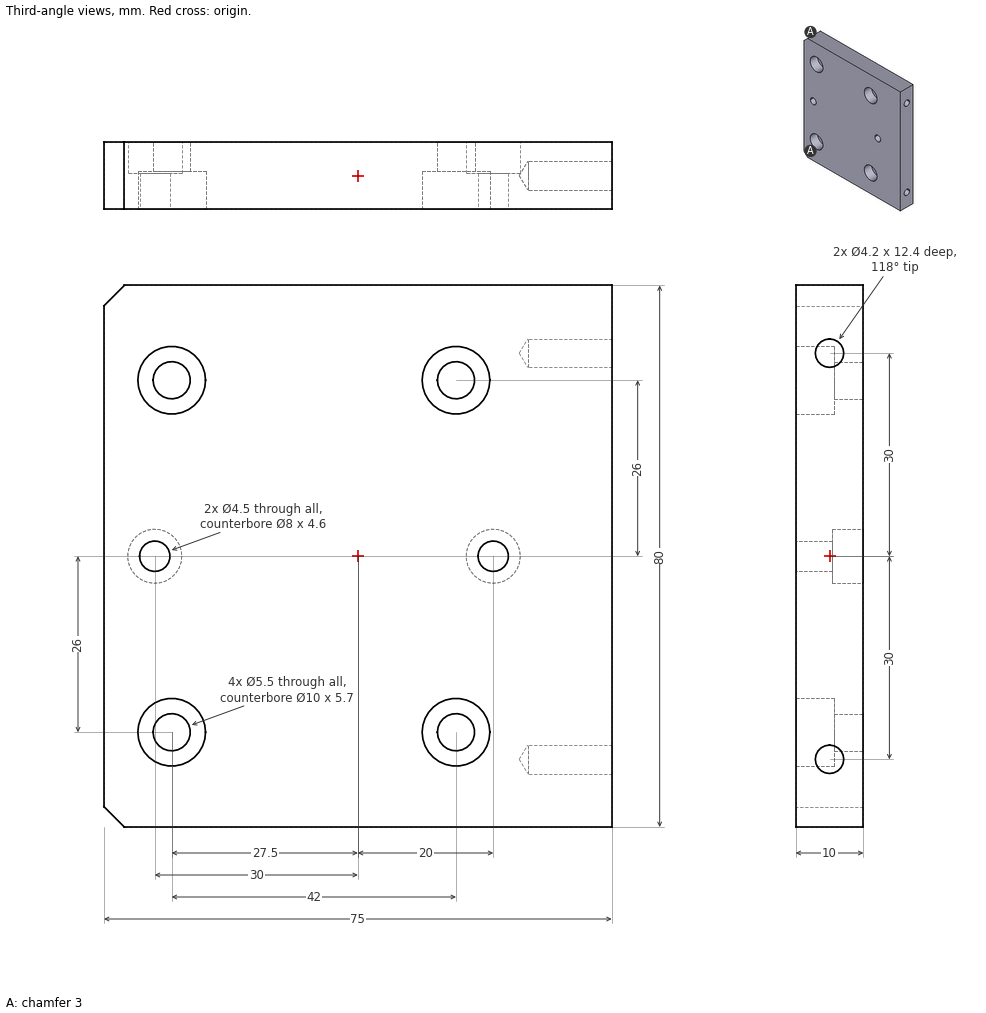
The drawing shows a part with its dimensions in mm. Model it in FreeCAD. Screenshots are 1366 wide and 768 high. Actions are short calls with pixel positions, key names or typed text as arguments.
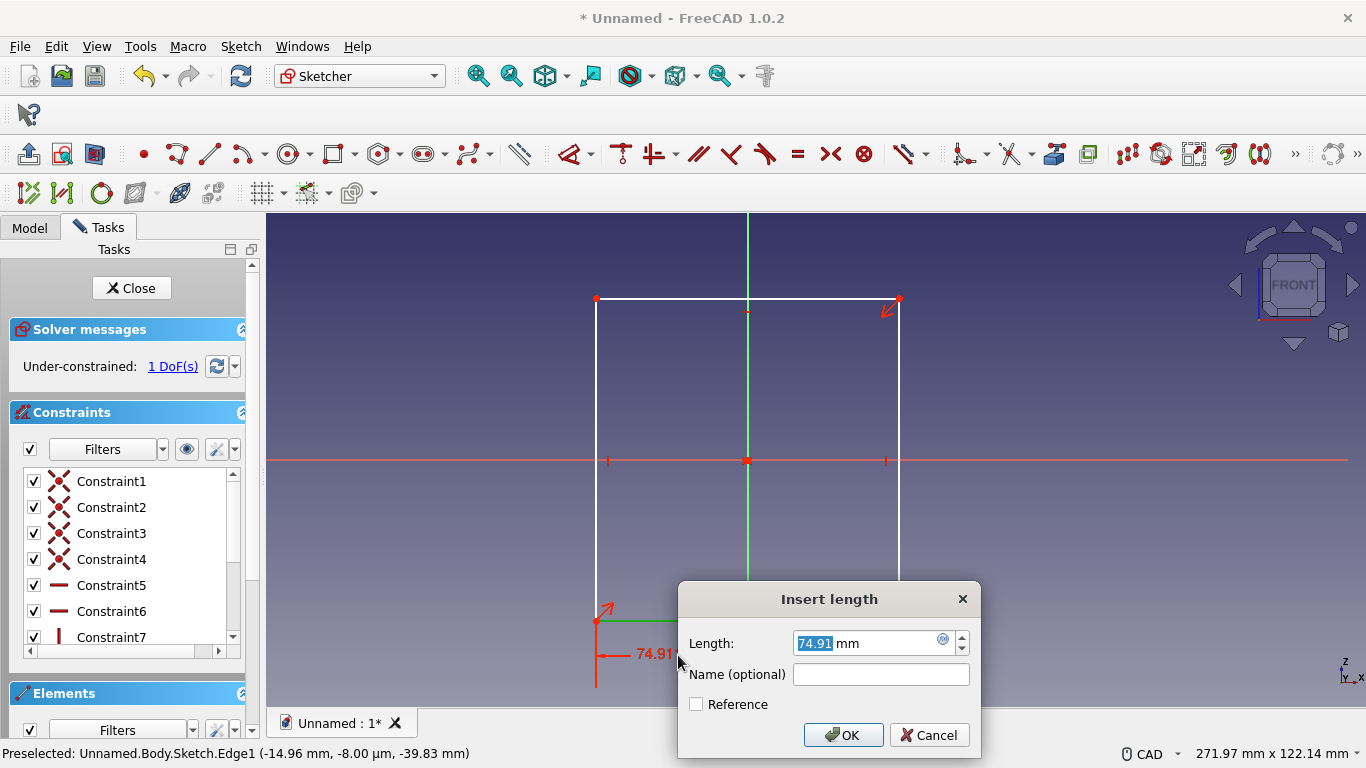
text(75)
key(Return)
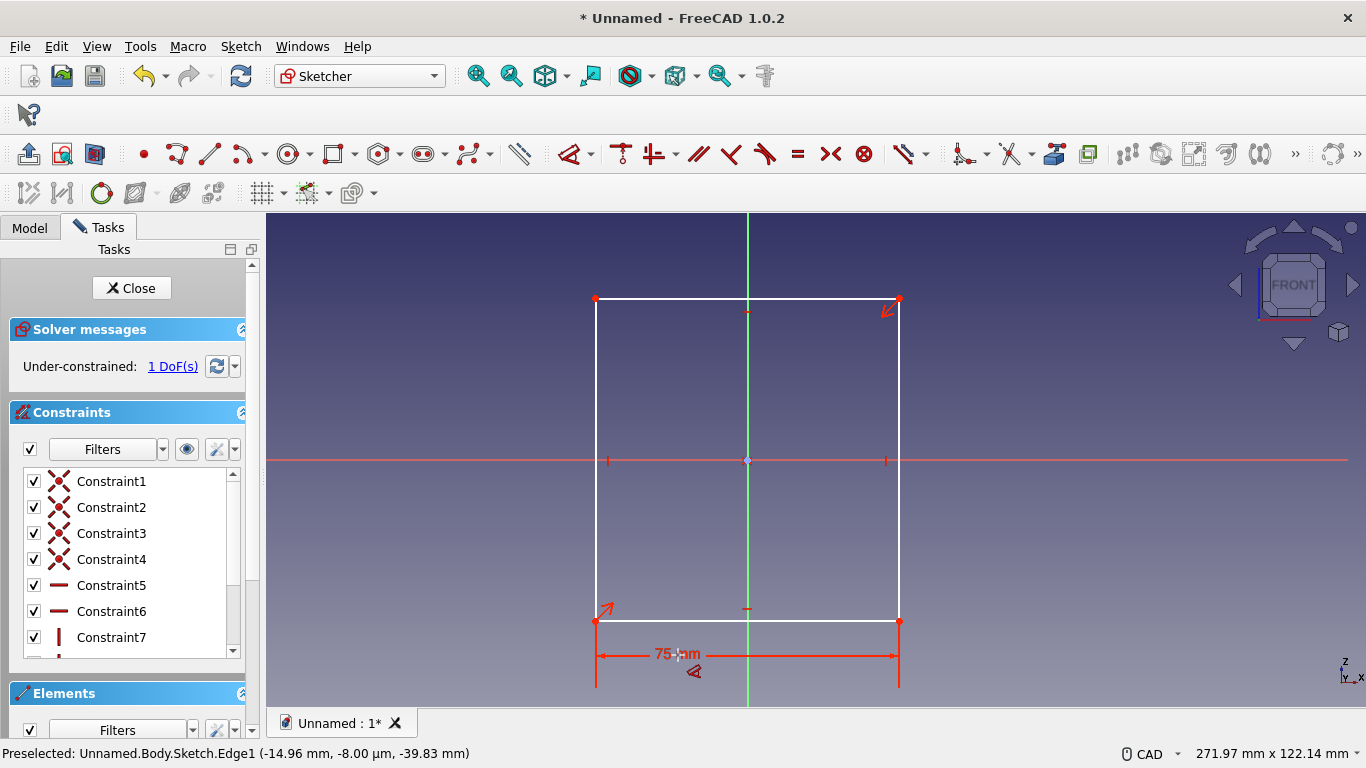
click(899, 525)
click(933, 386)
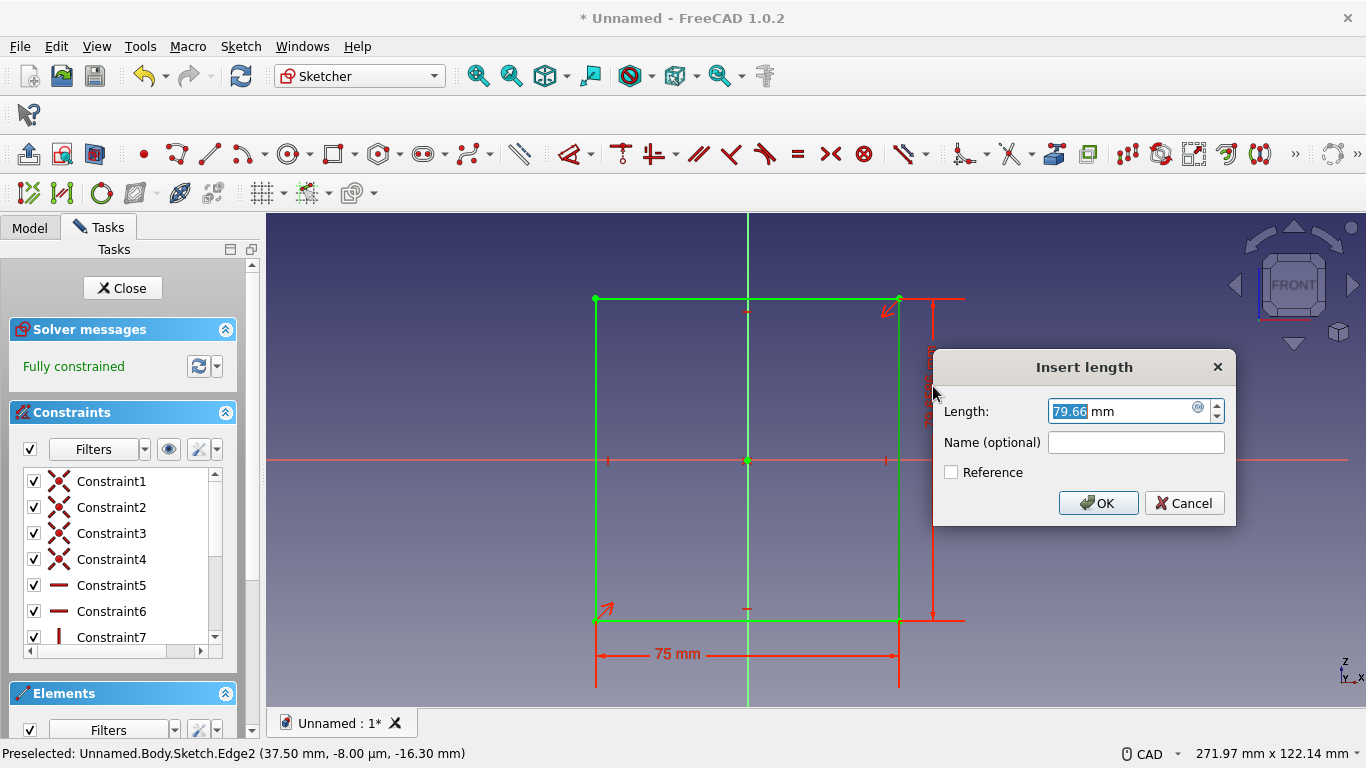
text(80)
key(Return)
key(Escape)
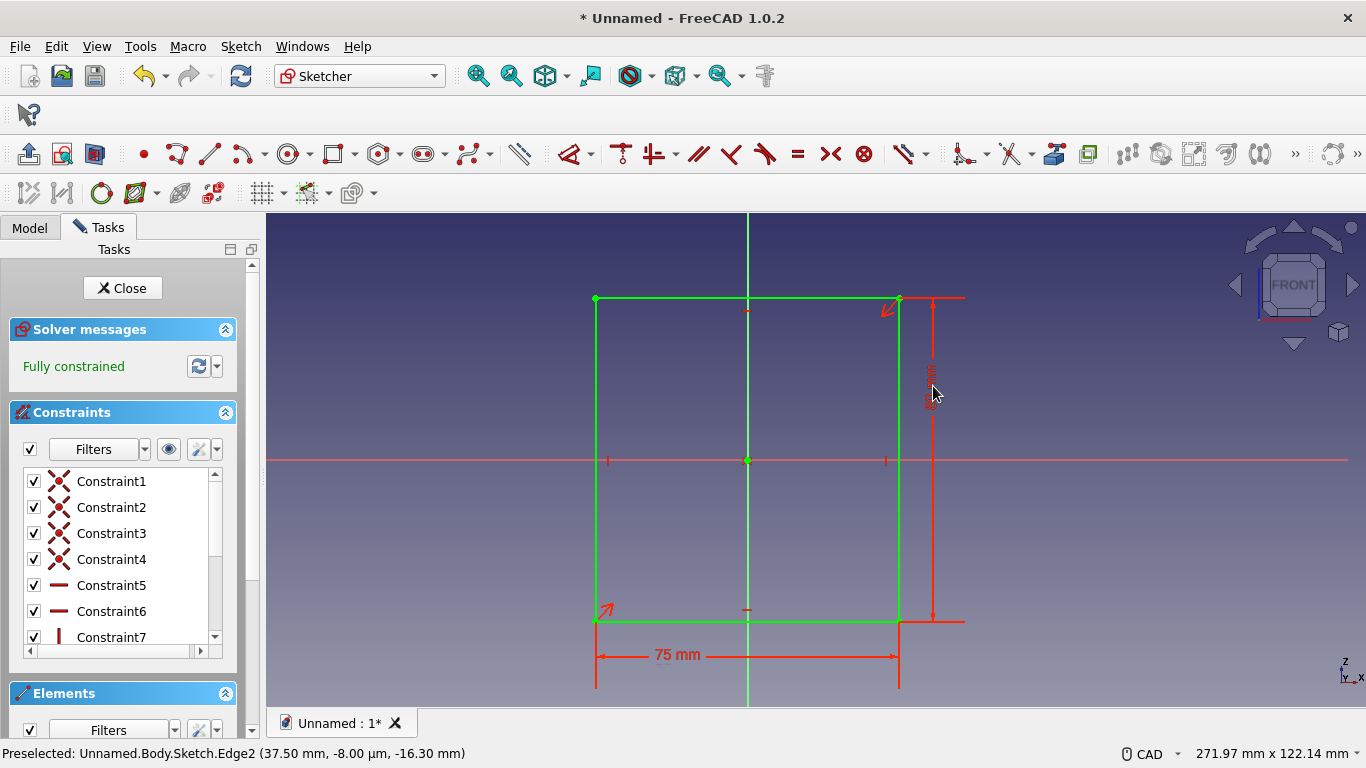
click(123, 288)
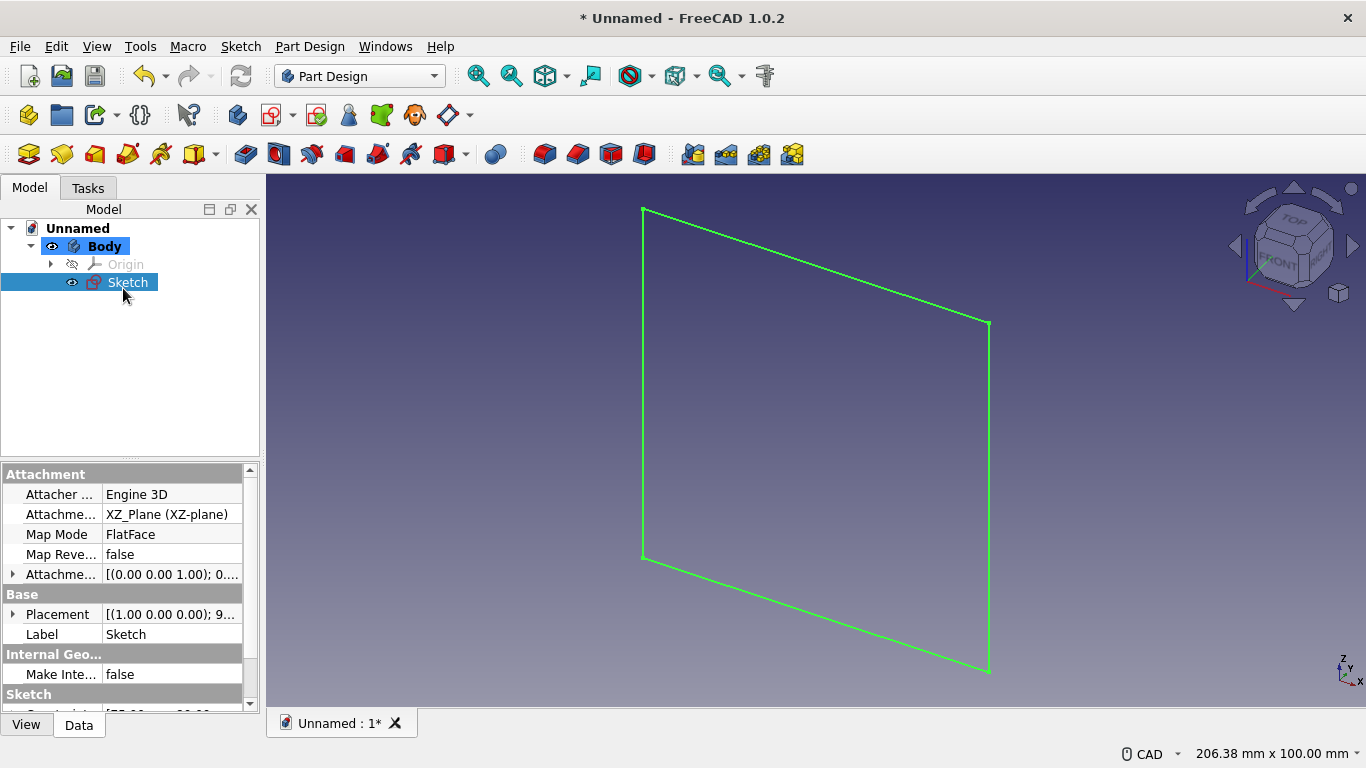
click(29, 154)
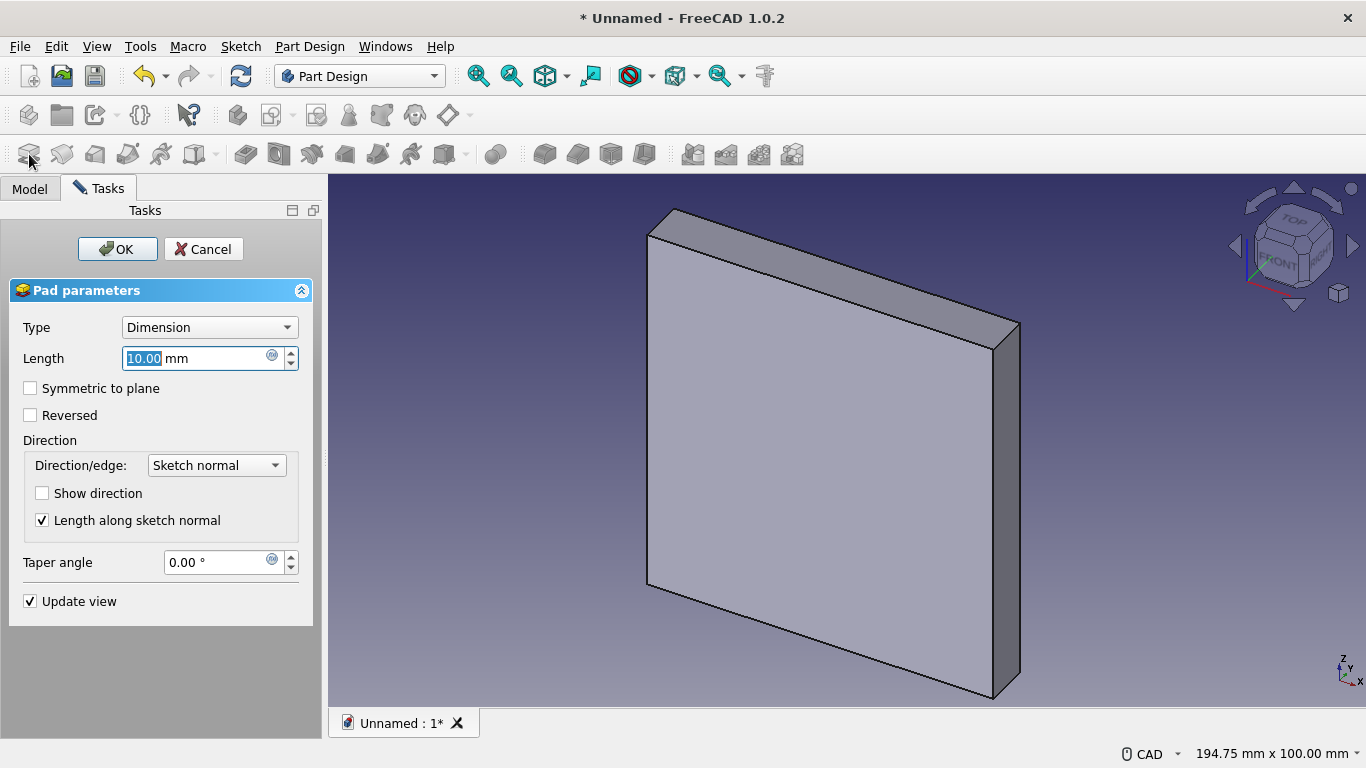
text(10)
key(Tab)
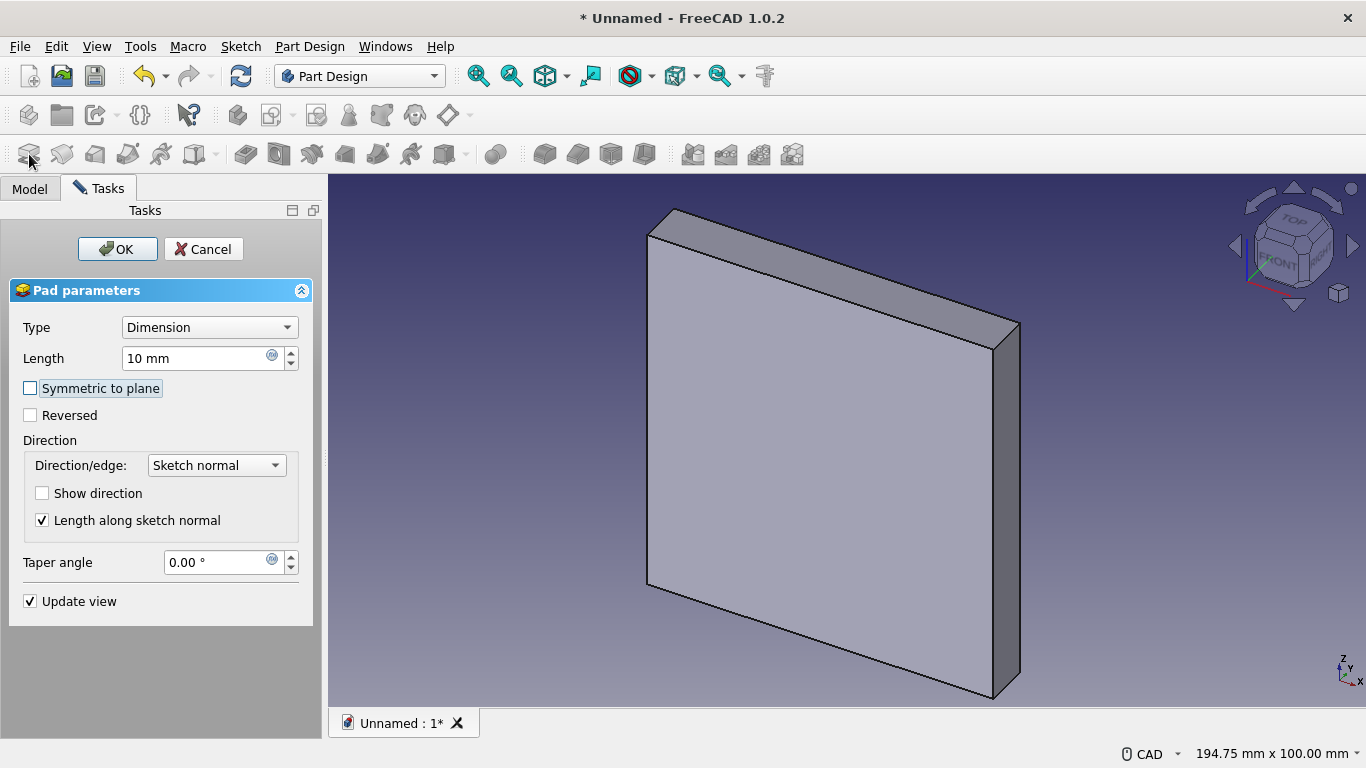
click(31, 388)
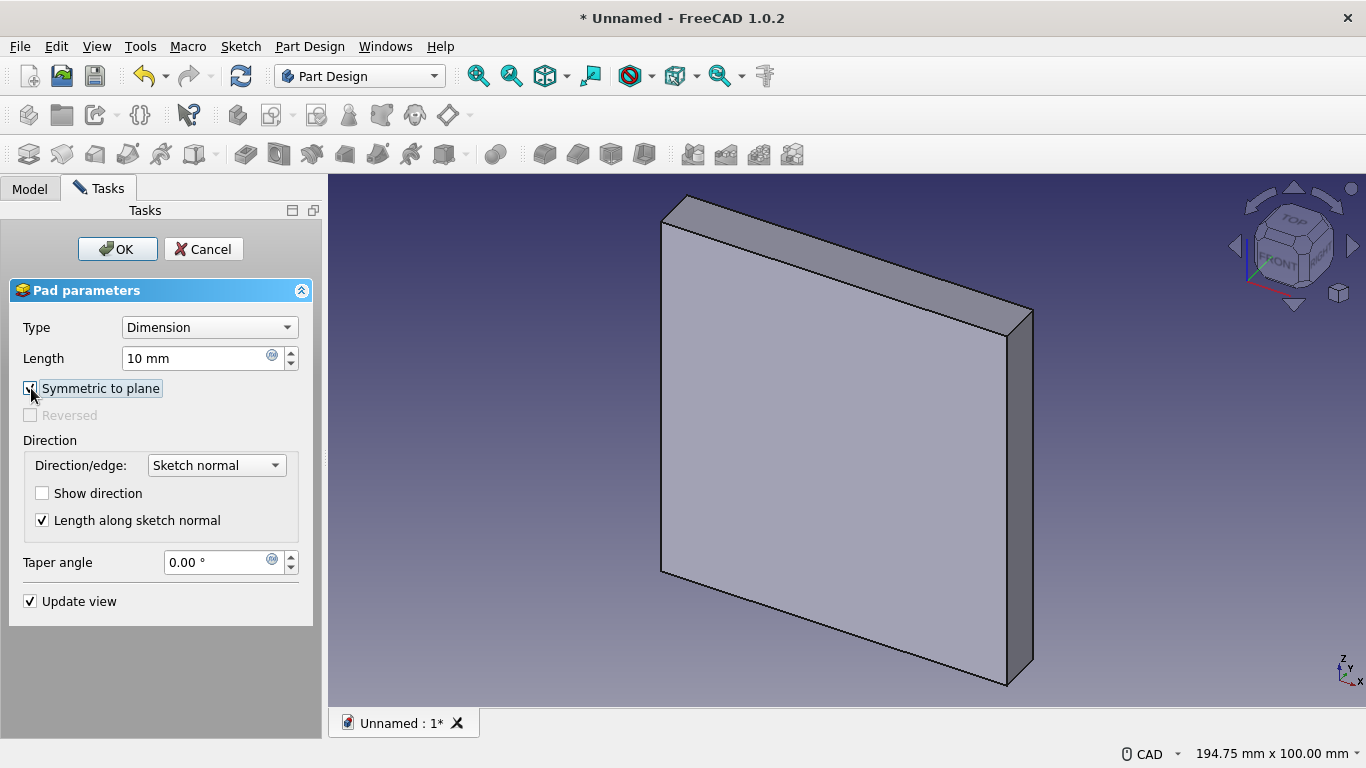
click(118, 249)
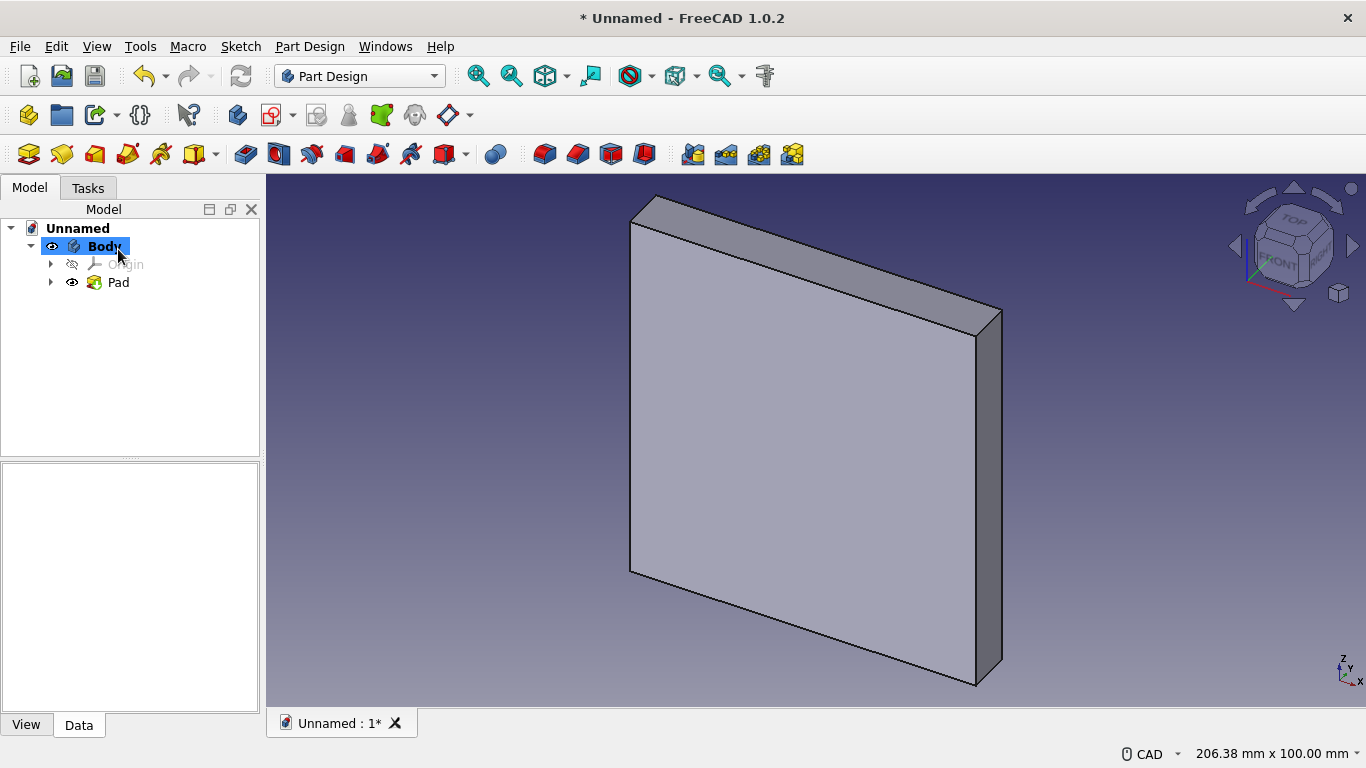
key(0)